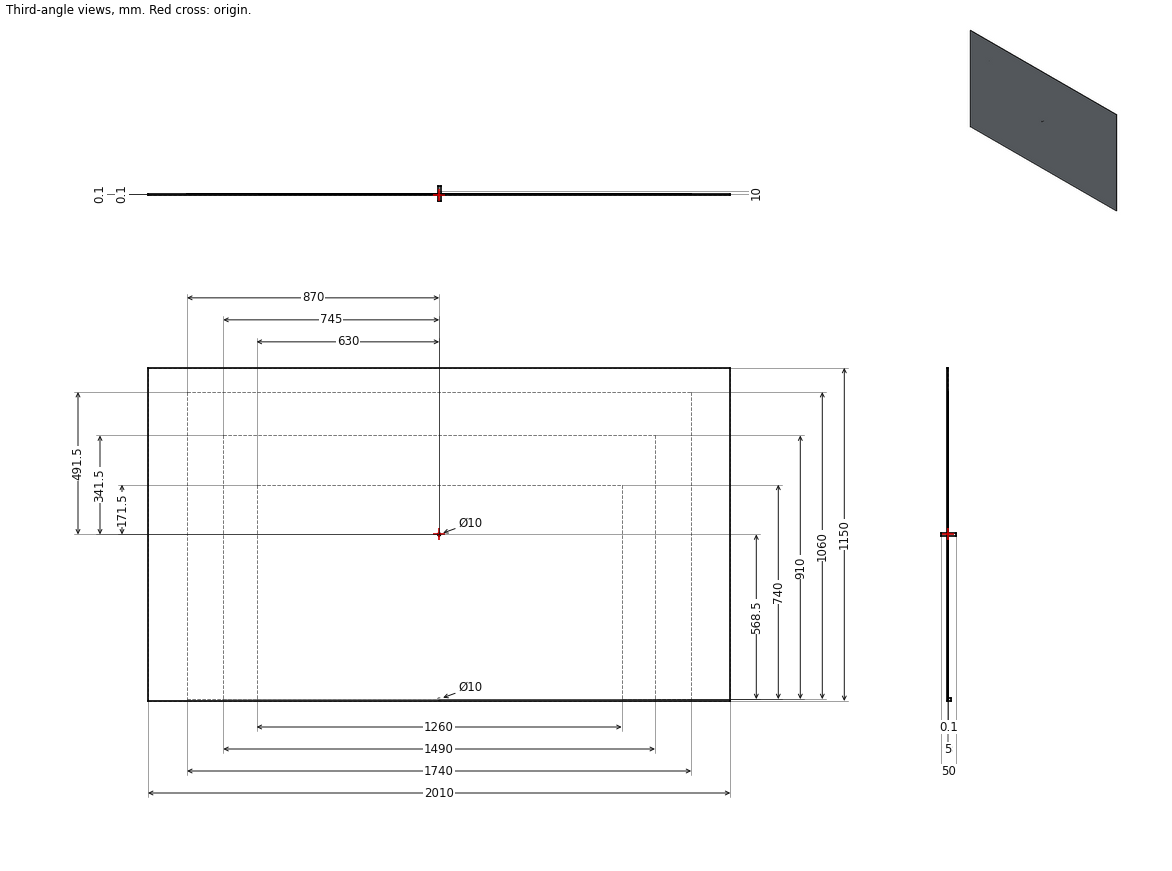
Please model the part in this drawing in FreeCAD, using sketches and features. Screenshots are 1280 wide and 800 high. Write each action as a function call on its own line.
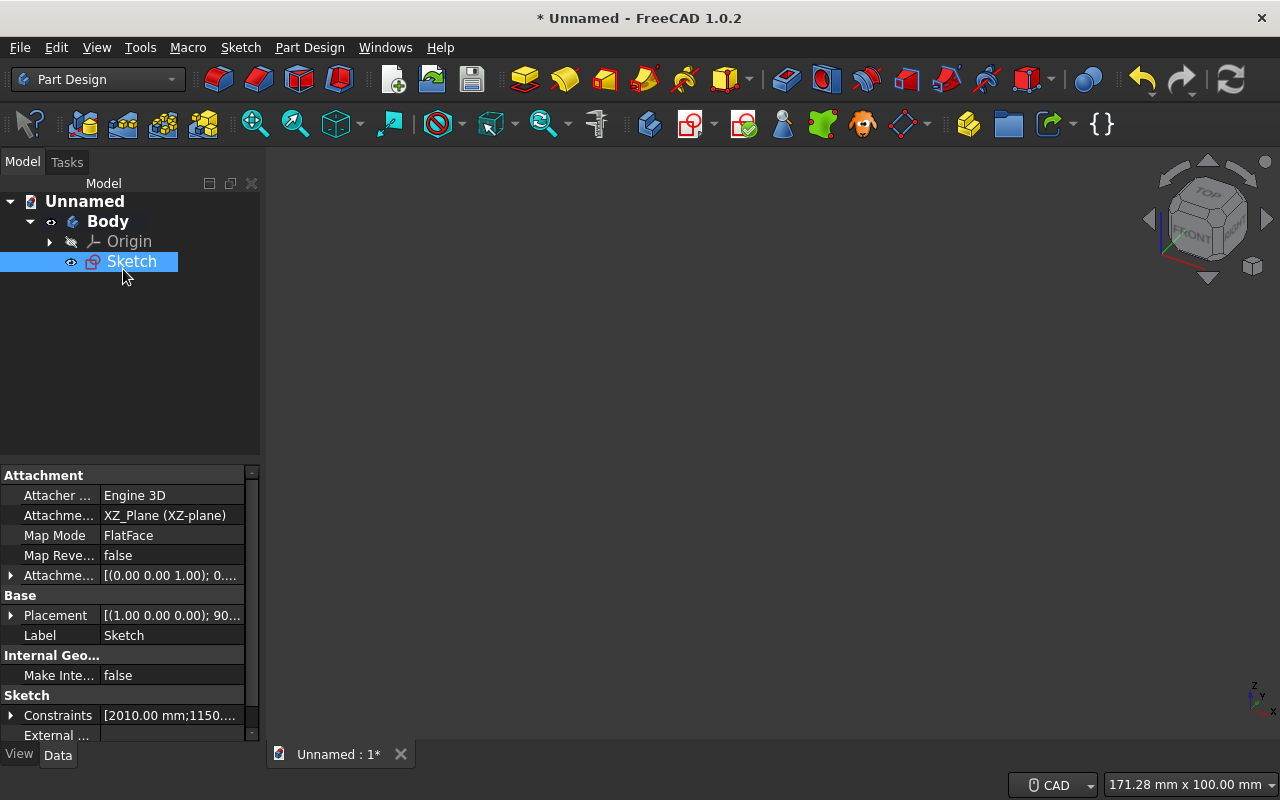
click(526, 80)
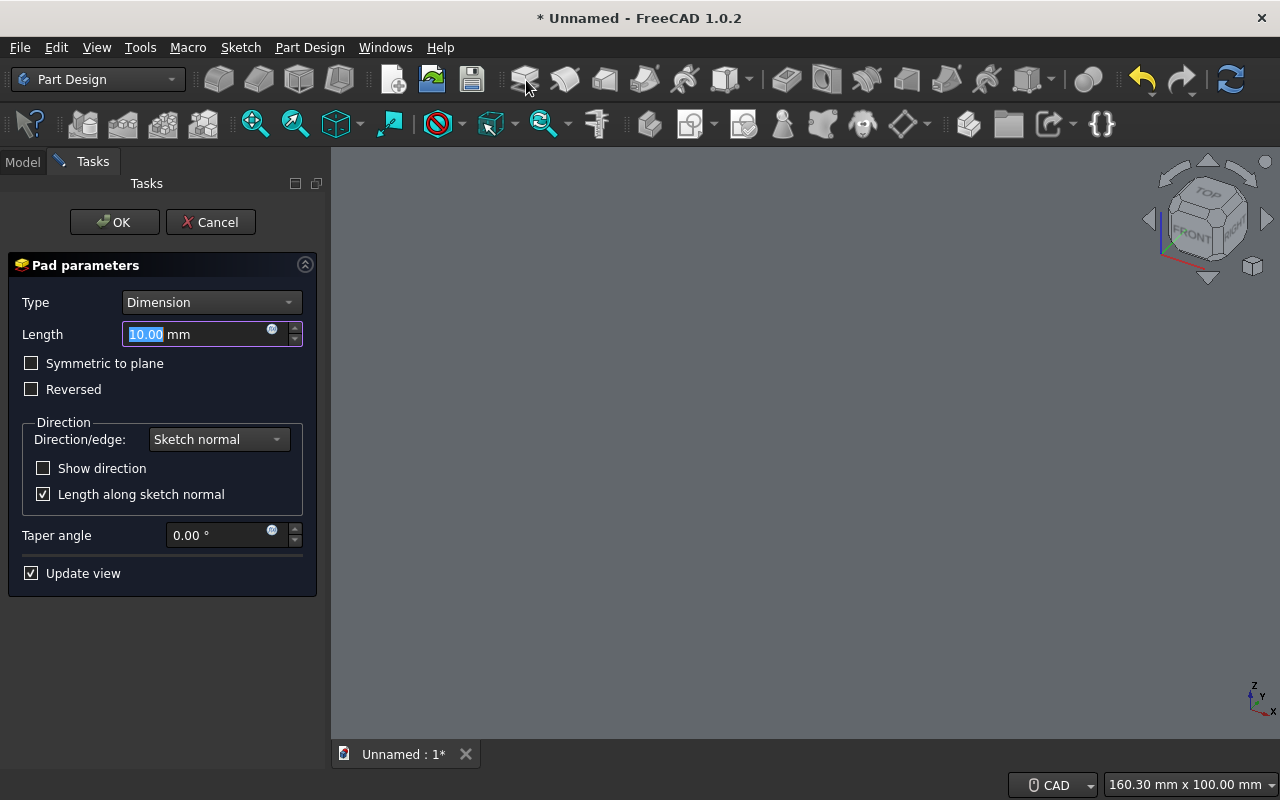
text(5)
key(Tab)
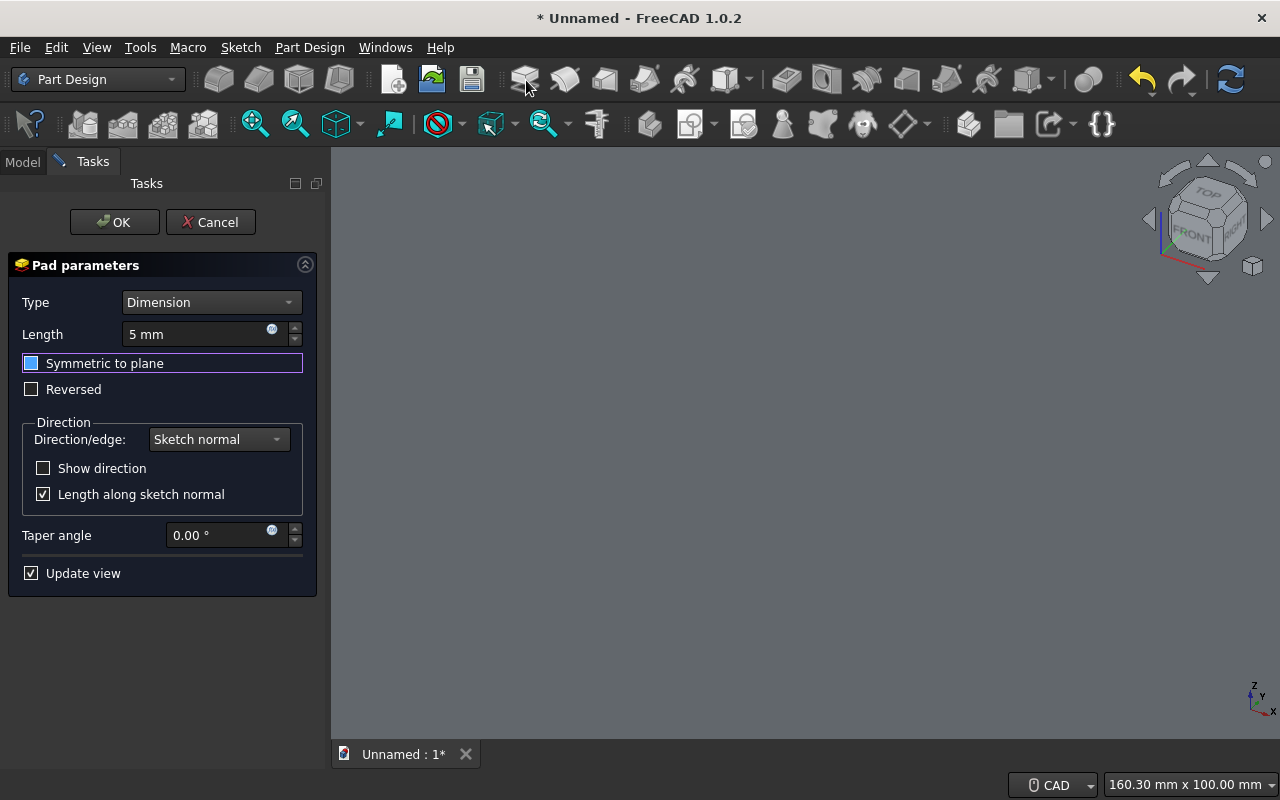
click(30, 363)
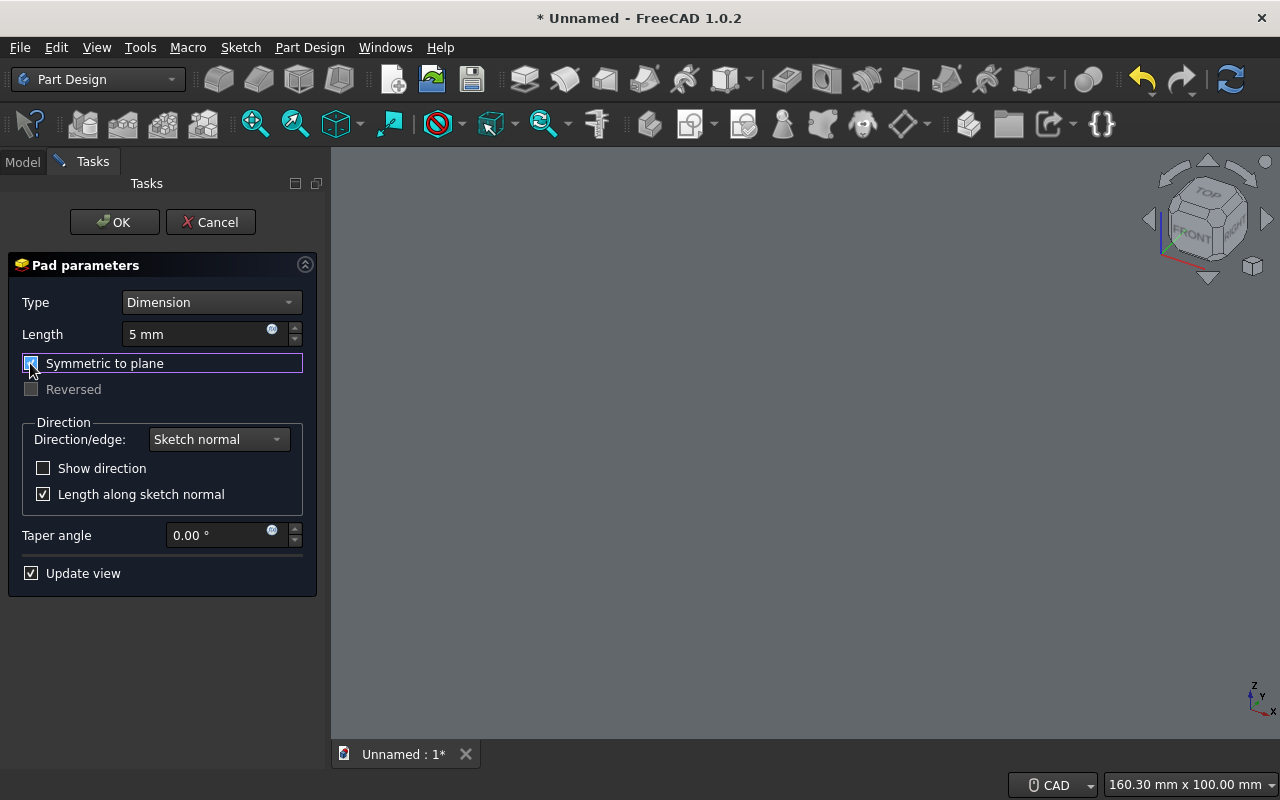
click(115, 222)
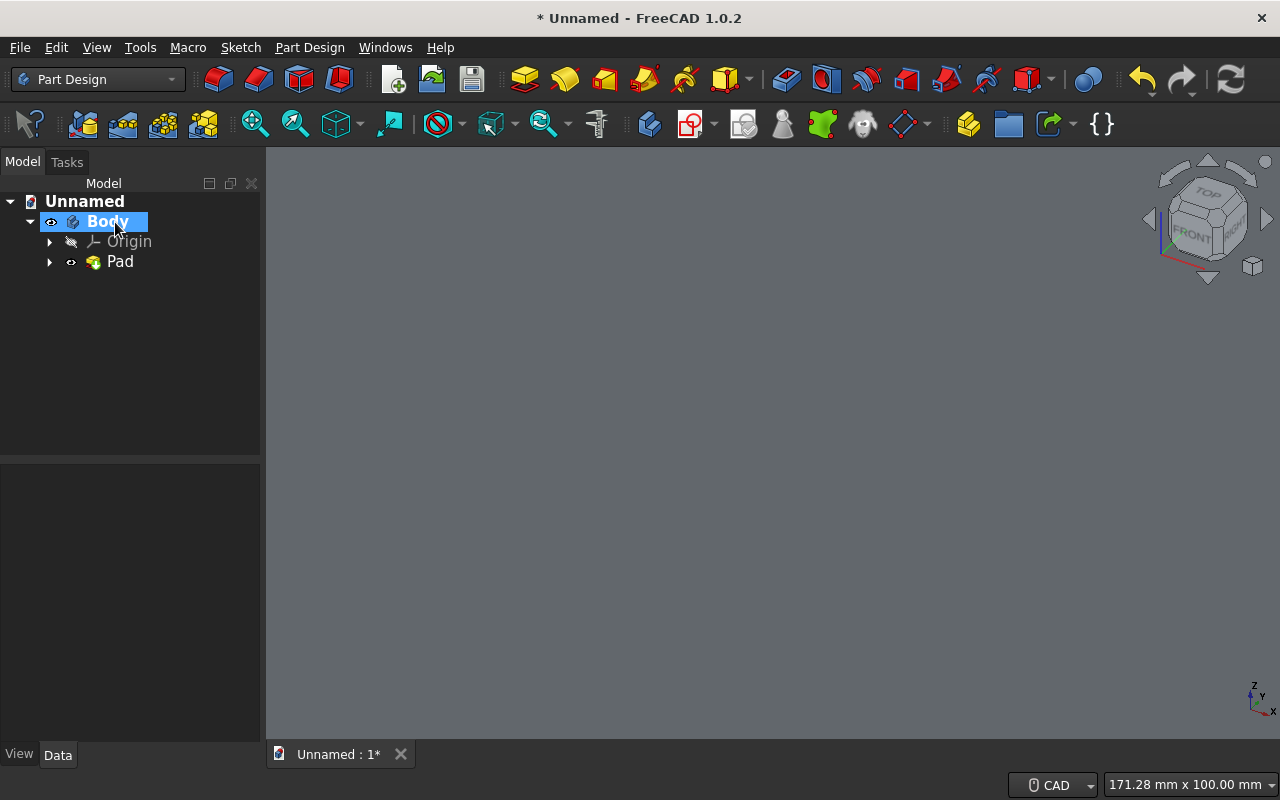
click(256, 124)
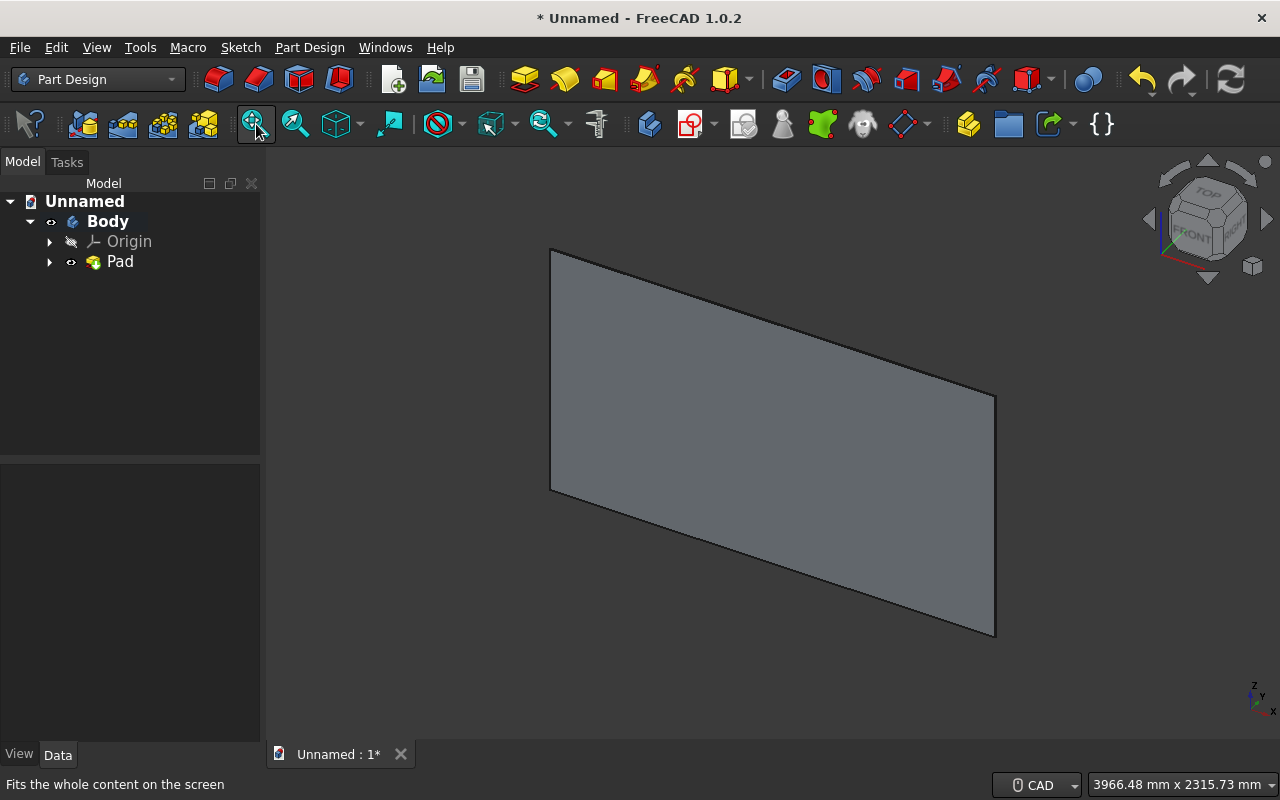
click(650, 124)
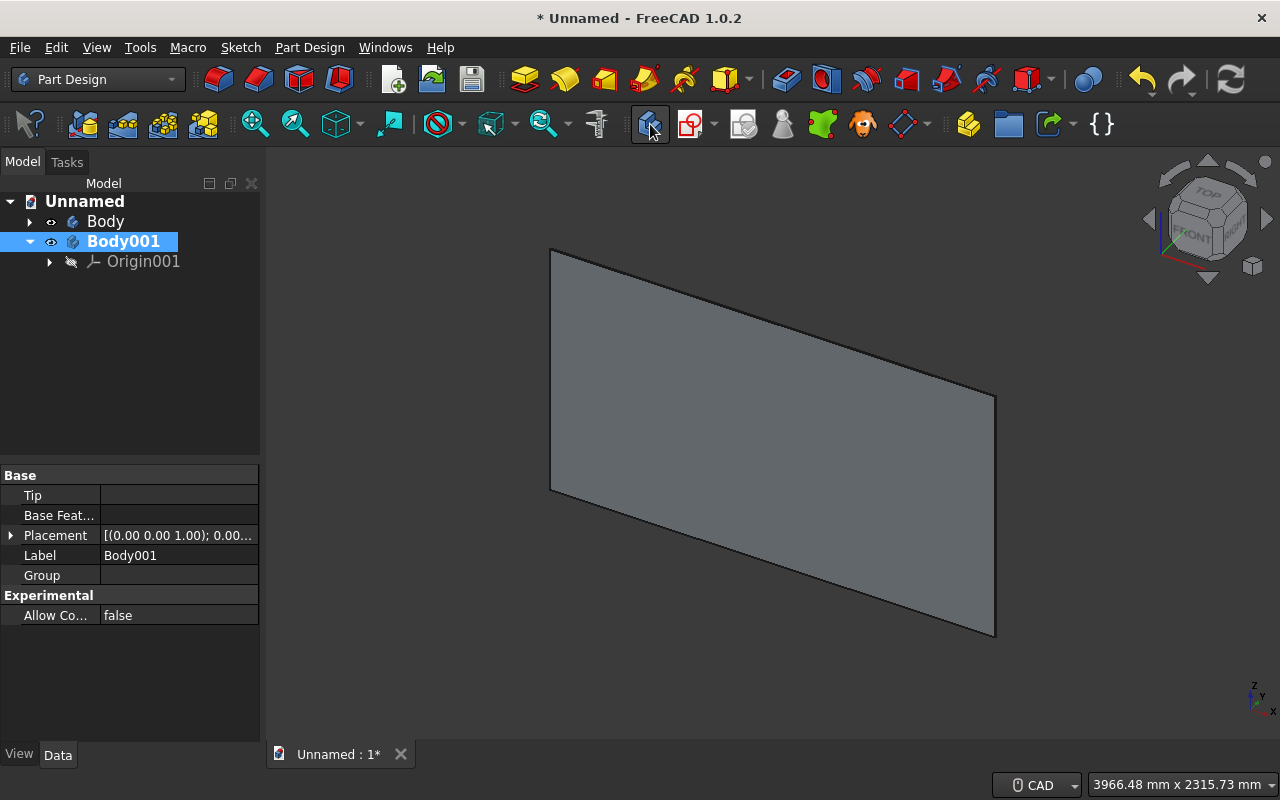
click(50, 262)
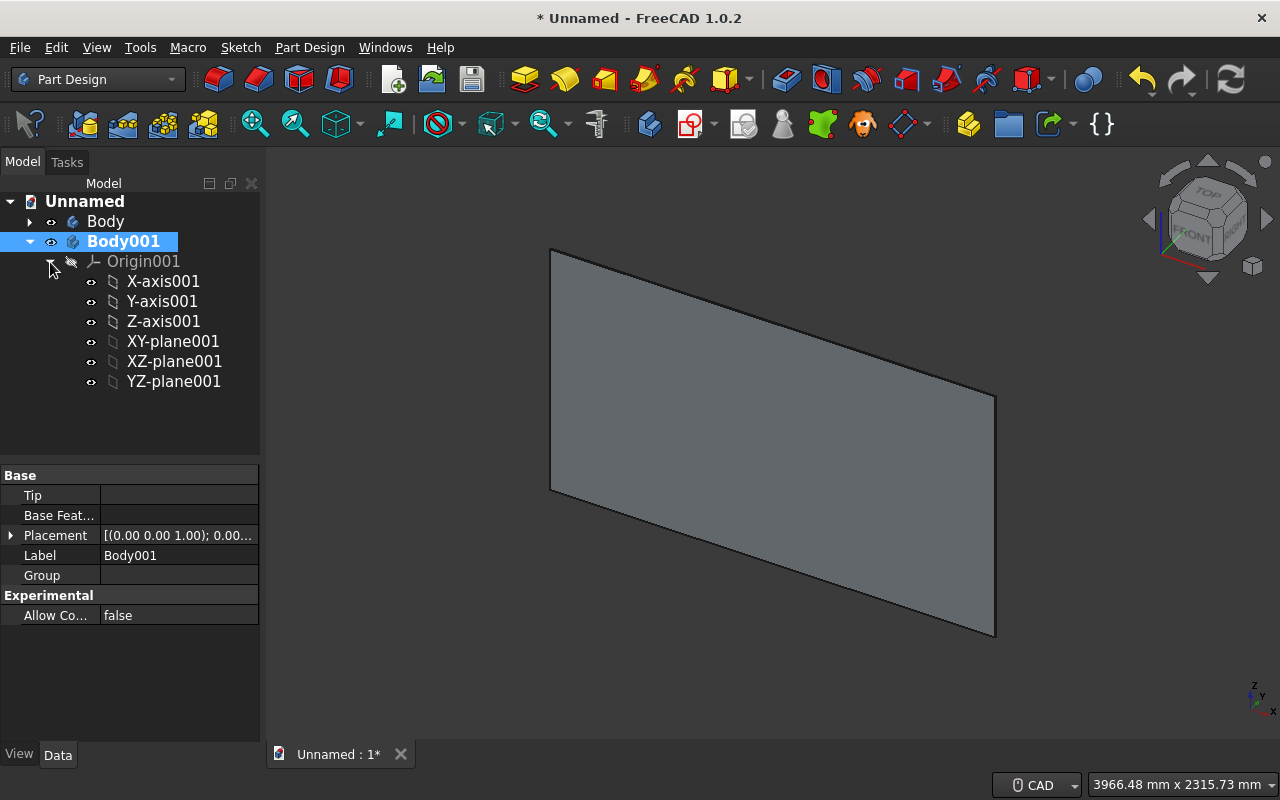
click(136, 362)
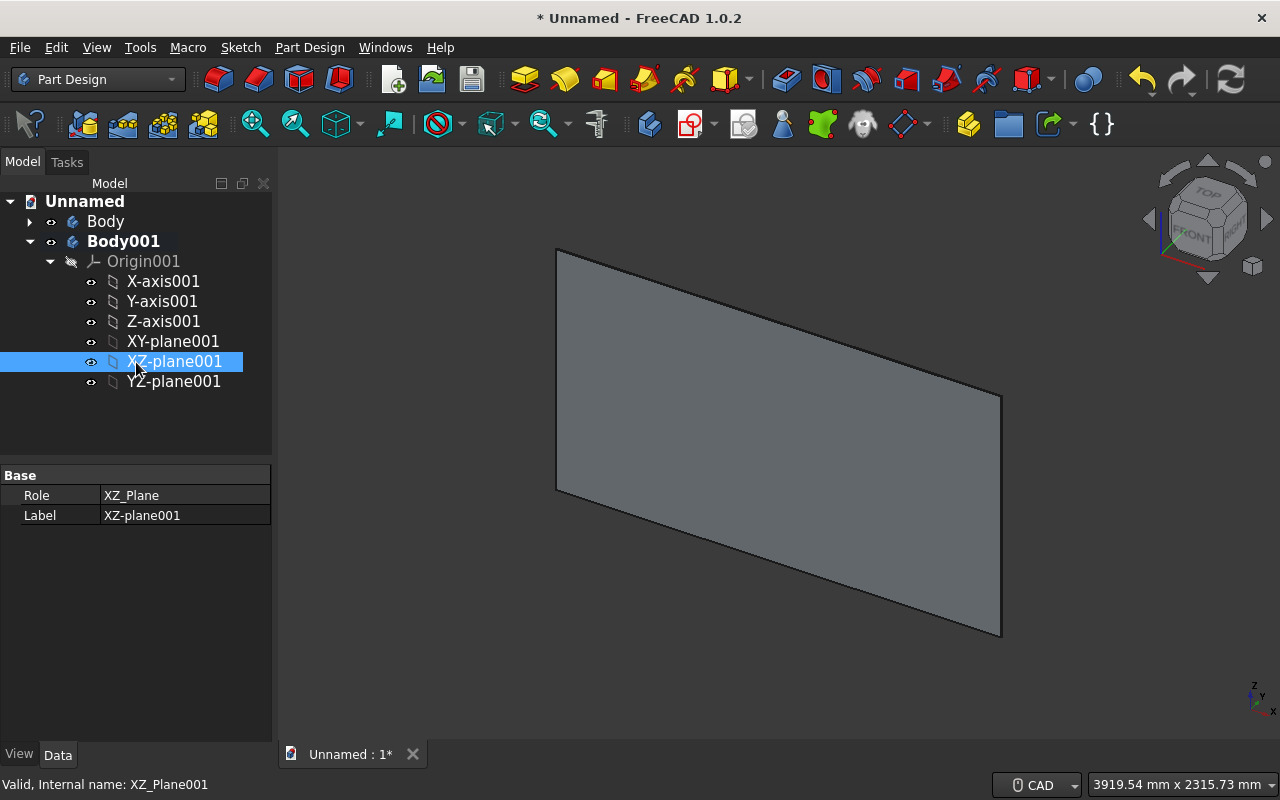
click(904, 124)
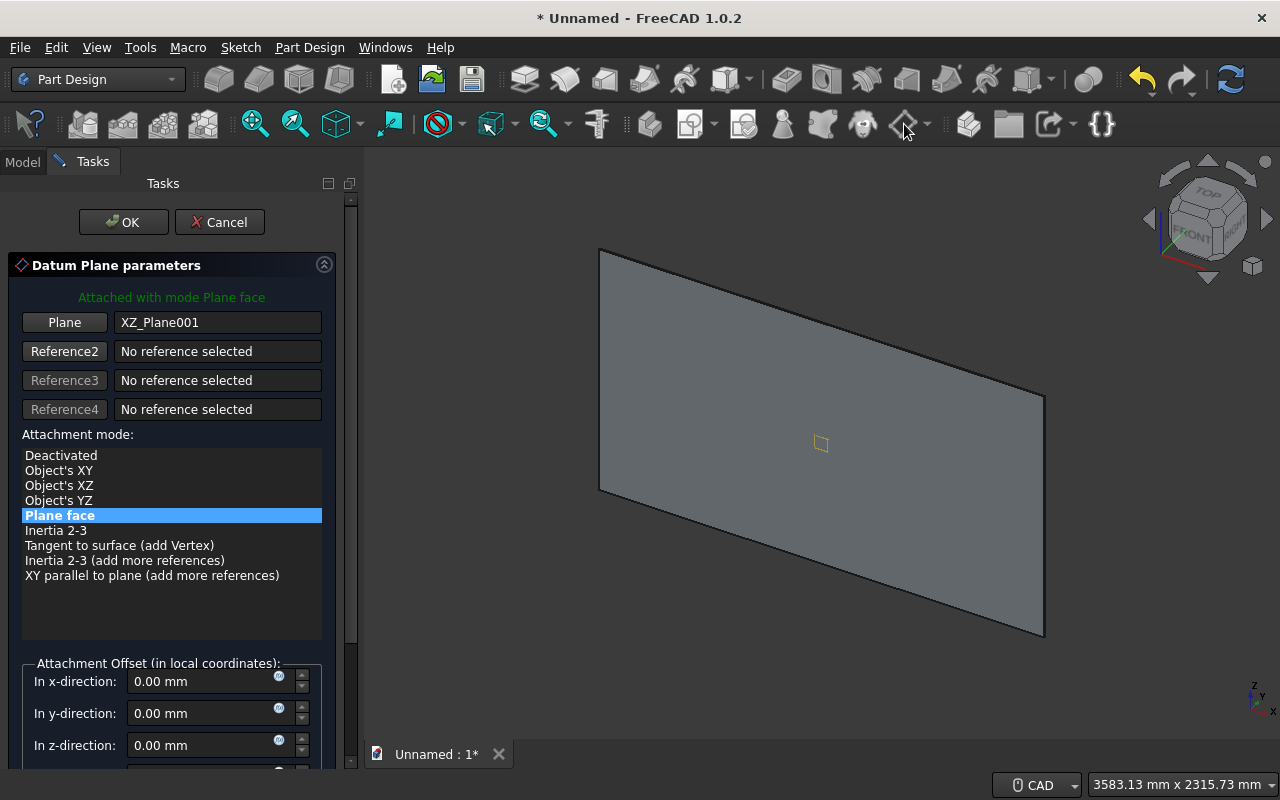
triple_click(210, 745)